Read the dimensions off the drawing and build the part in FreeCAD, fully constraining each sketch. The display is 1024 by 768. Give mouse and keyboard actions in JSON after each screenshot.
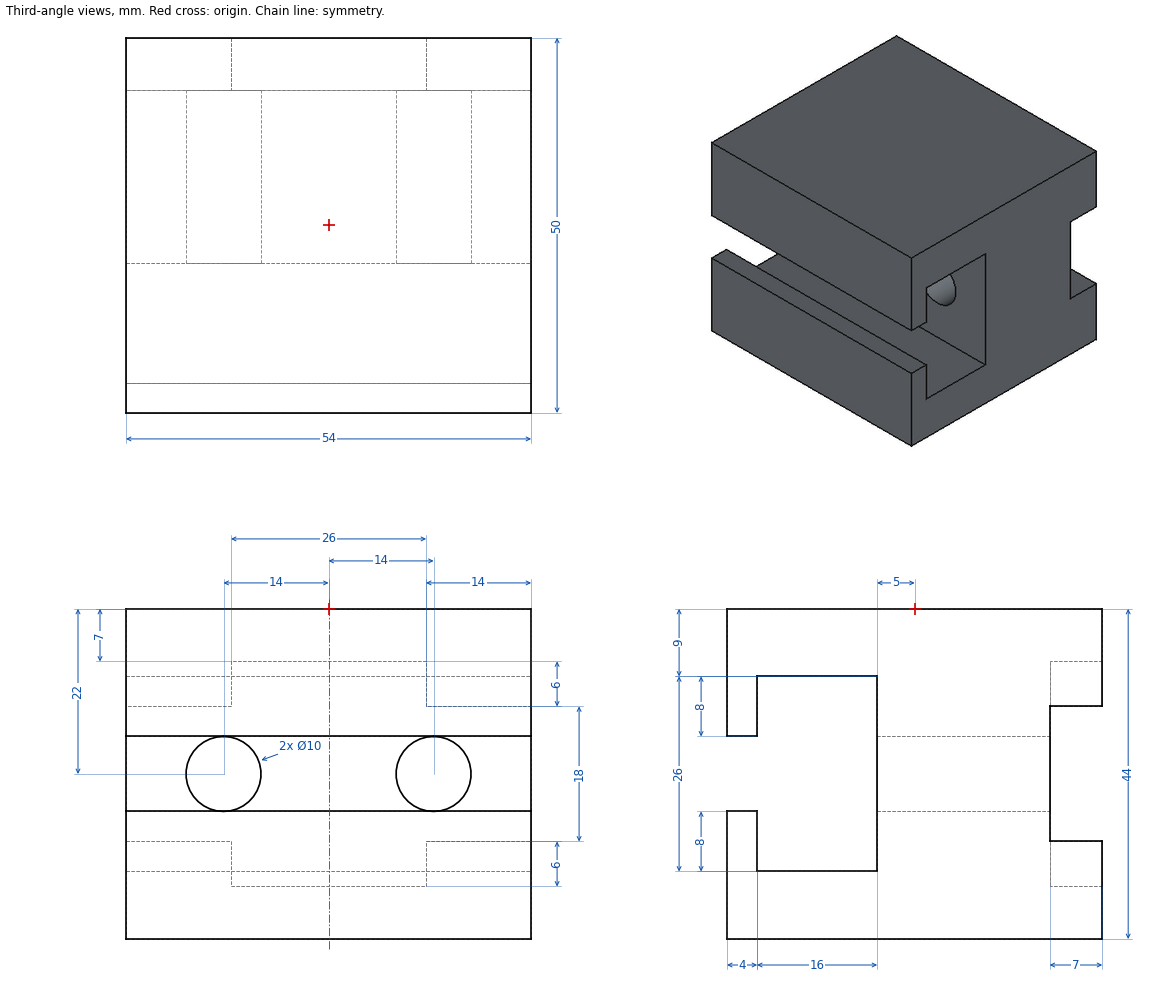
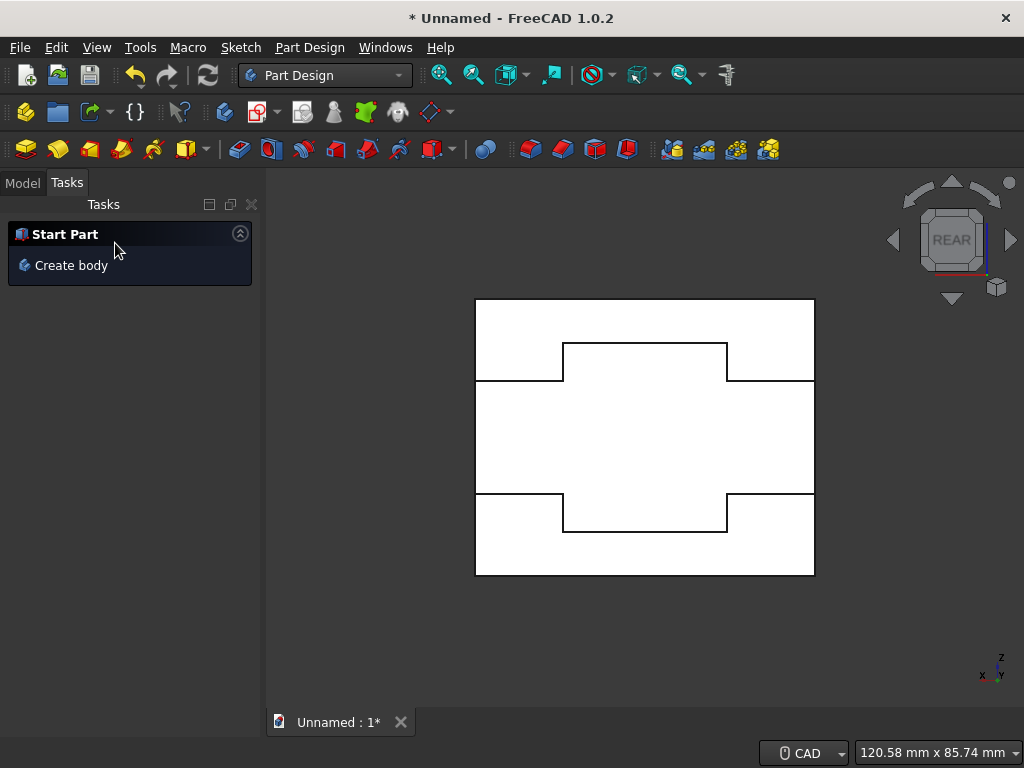
{"action": "key", "text": "6"}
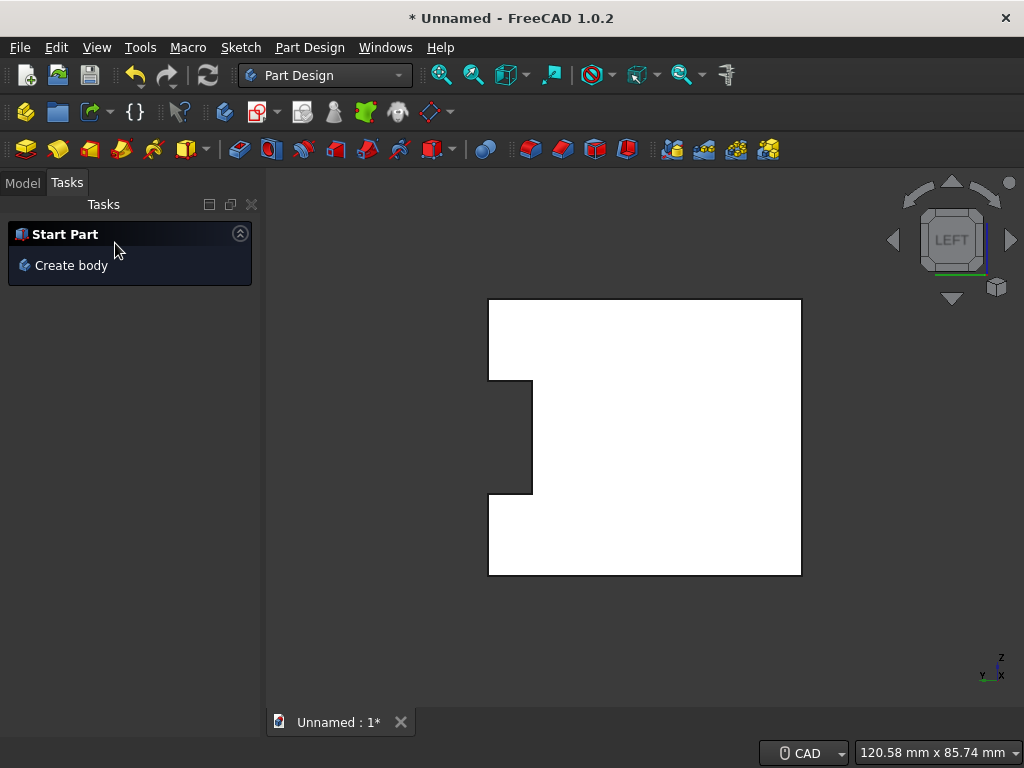
{"action": "left_click", "coordinate": [645, 437]}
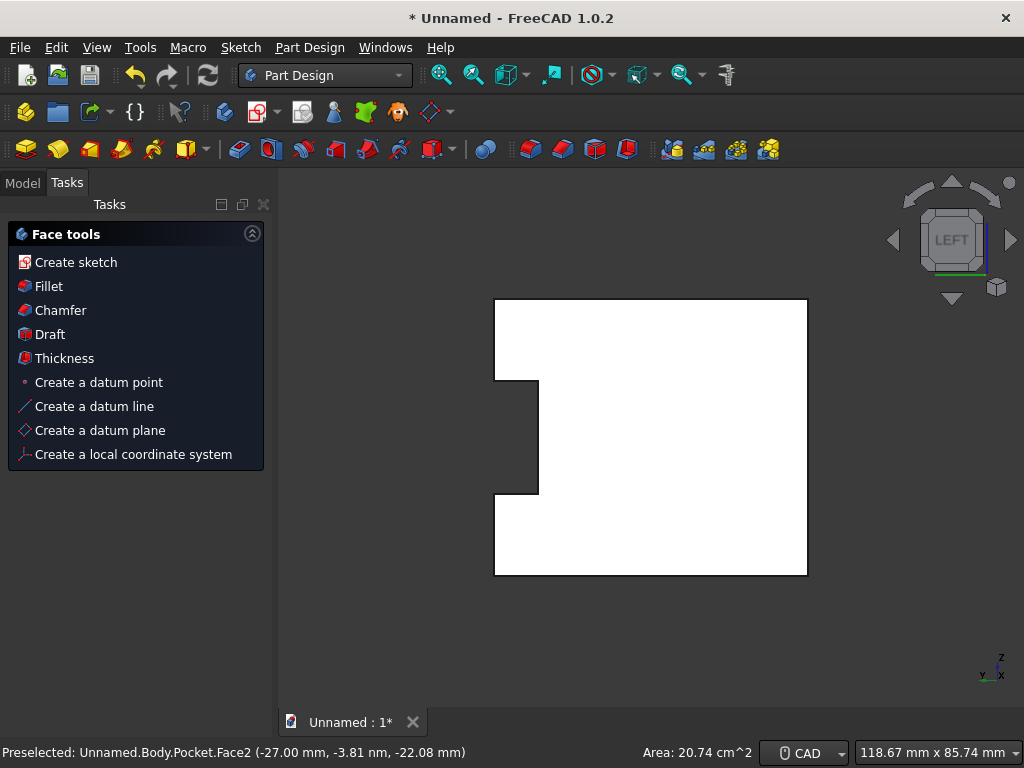
{"action": "left_click", "coordinate": [258, 112]}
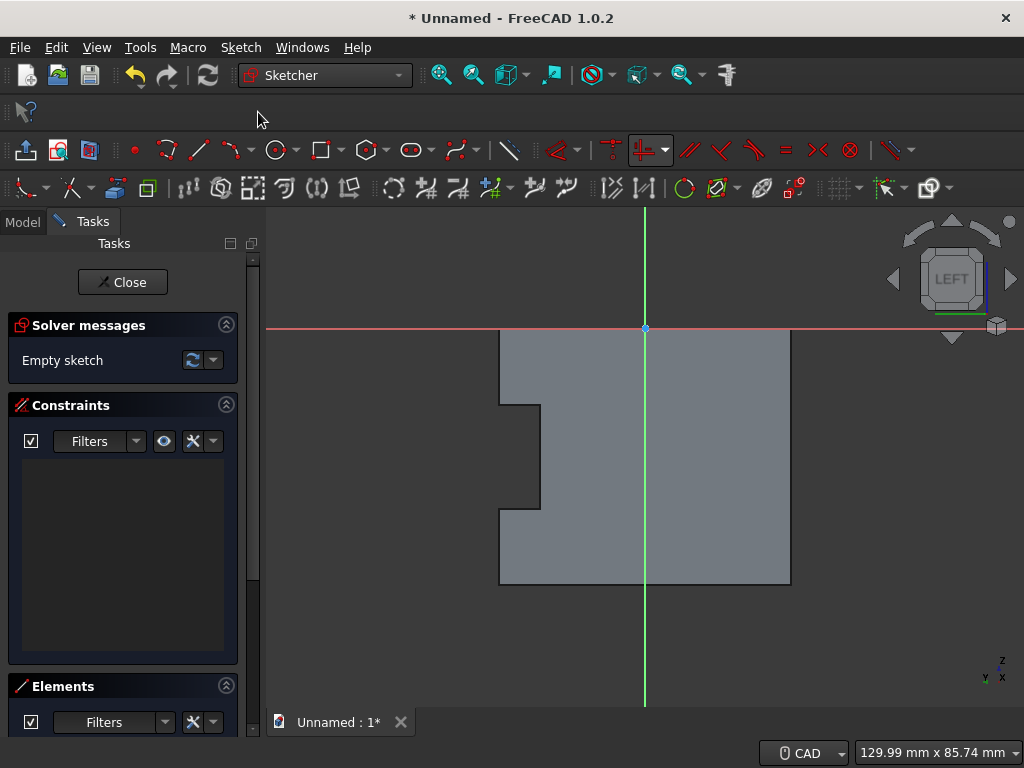
{"action": "scroll", "coordinate": [859, 377], "scroll_direction": "up", "scroll_amount": 2}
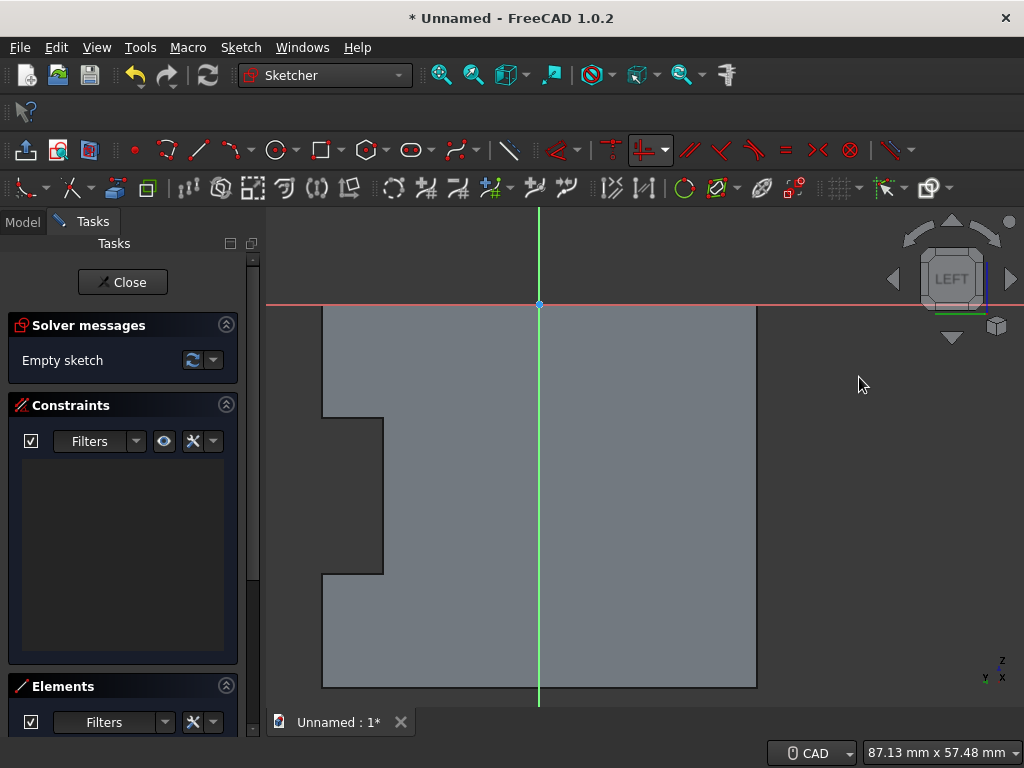
{"action": "left_click", "coordinate": [168, 150]}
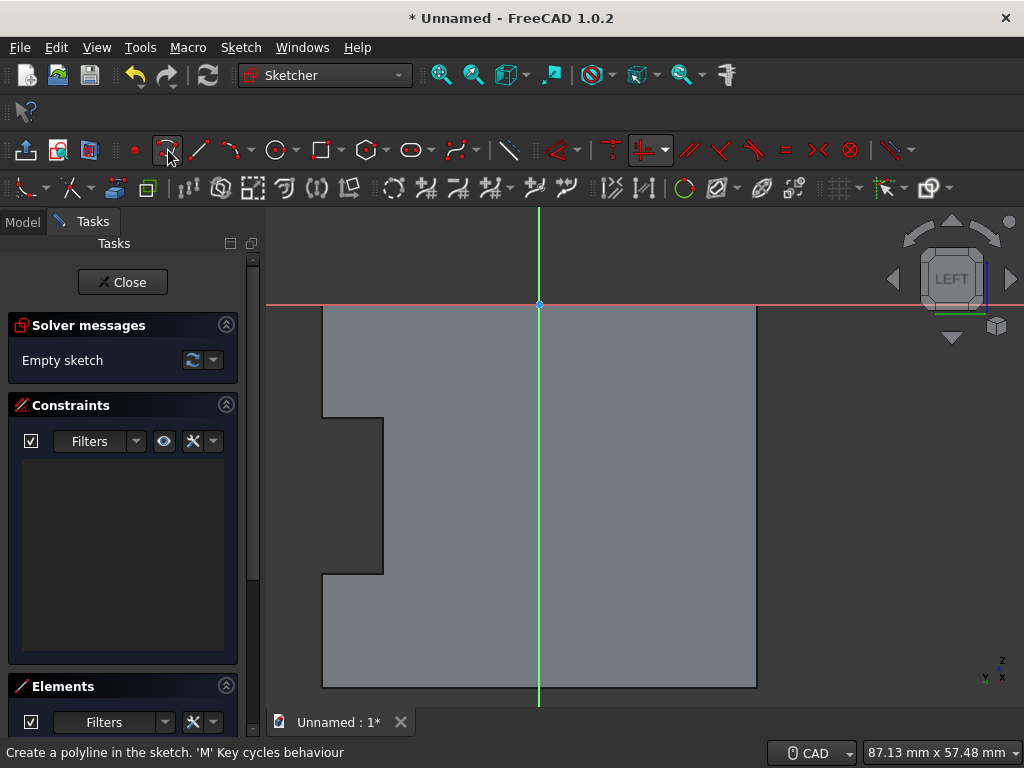
{"action": "left_click", "coordinate": [583, 383]}
{"action": "left_click", "coordinate": [583, 609]}
{"action": "left_click", "coordinate": [722, 609]}
{"action": "left_click", "coordinate": [722, 540]}
{"action": "left_click", "coordinate": [757, 540]}
{"action": "left_click", "coordinate": [757, 453]}
{"action": "left_click", "coordinate": [722, 453]}
{"action": "left_click", "coordinate": [722, 383]}
{"action": "left_click", "coordinate": [583, 384]}
{"action": "key", "text": "Escape"}
{"action": "key", "text": "Escape"}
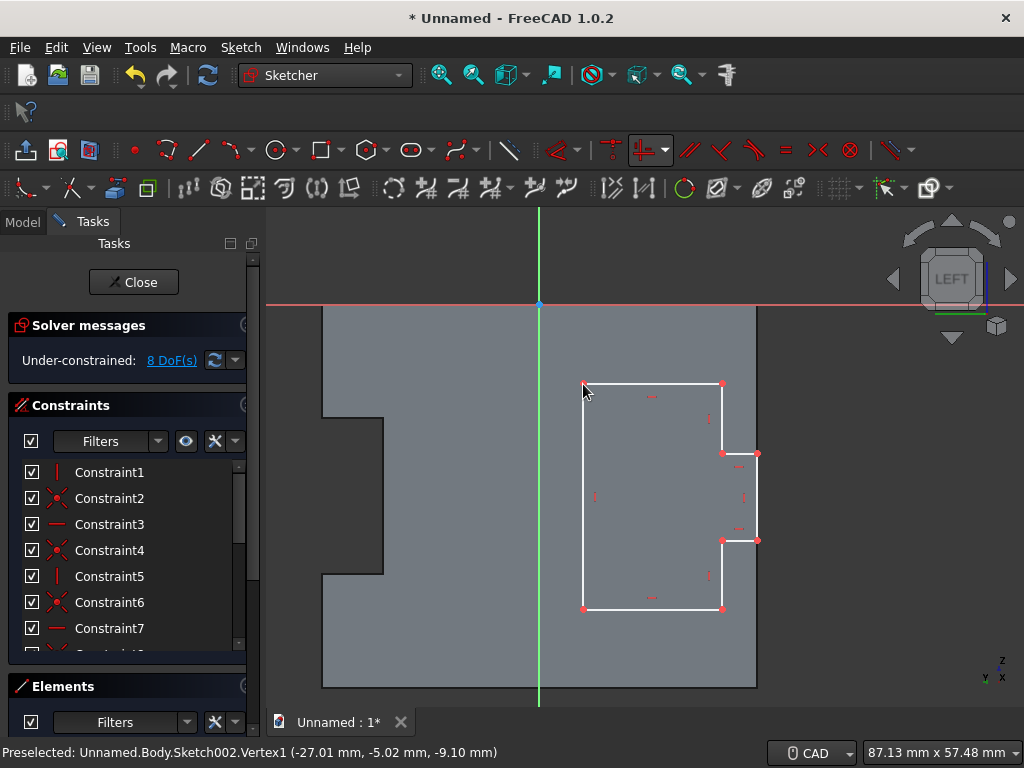
{"action": "key", "text": "d"}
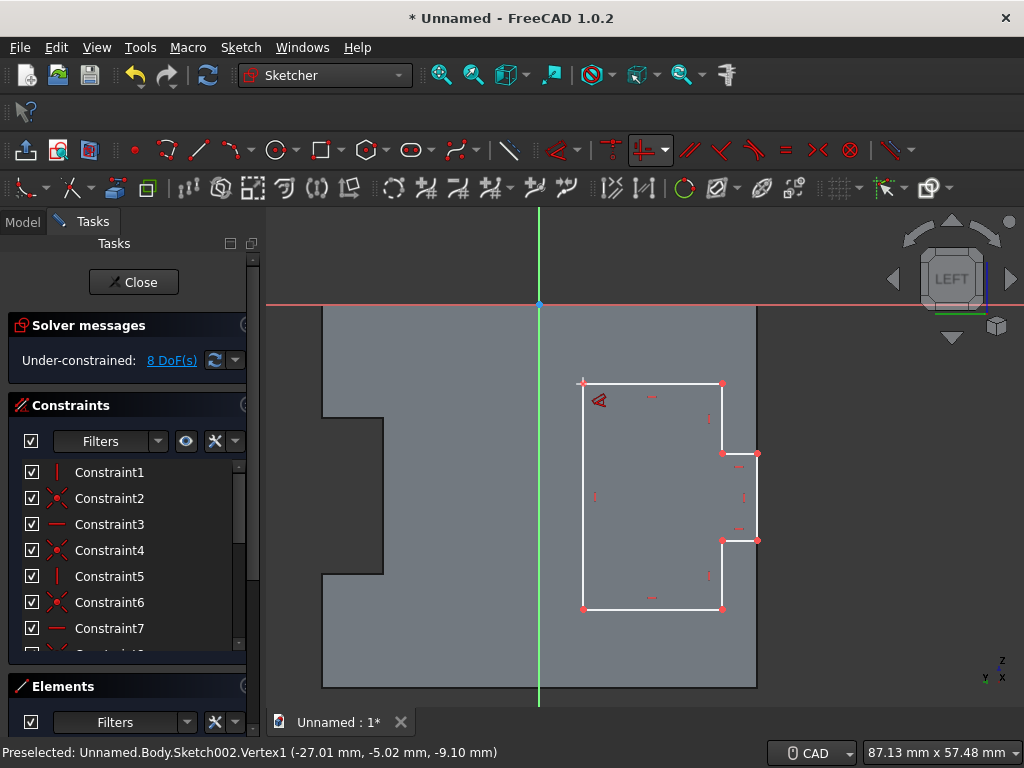
{"action": "left_click", "coordinate": [722, 589]}
{"action": "left_click", "coordinate": [756, 575]}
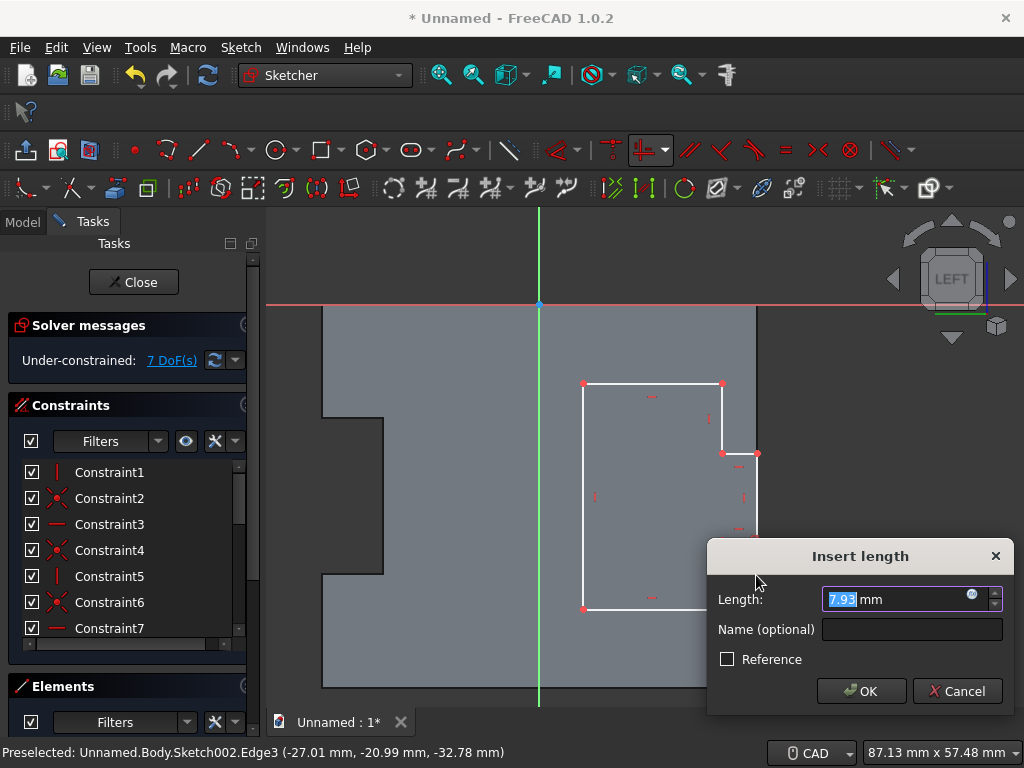
{"action": "type", "text": "8"}
{"action": "key", "text": "Return"}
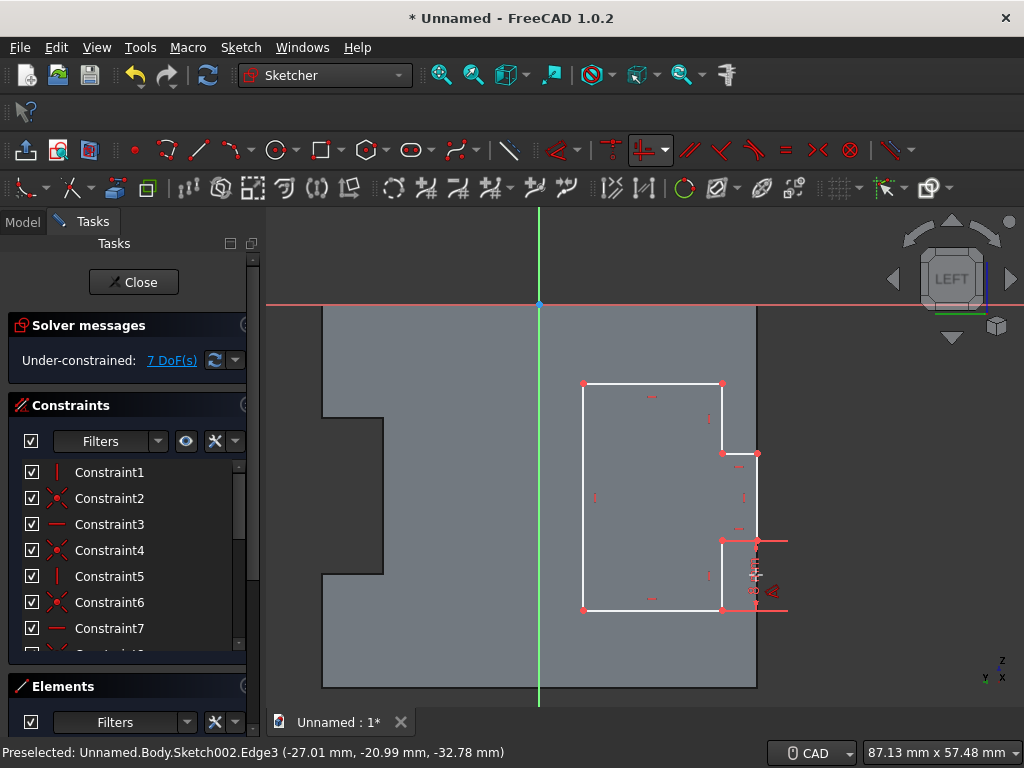
{"action": "scroll", "coordinate": [733, 541], "scroll_direction": "up", "scroll_amount": 2}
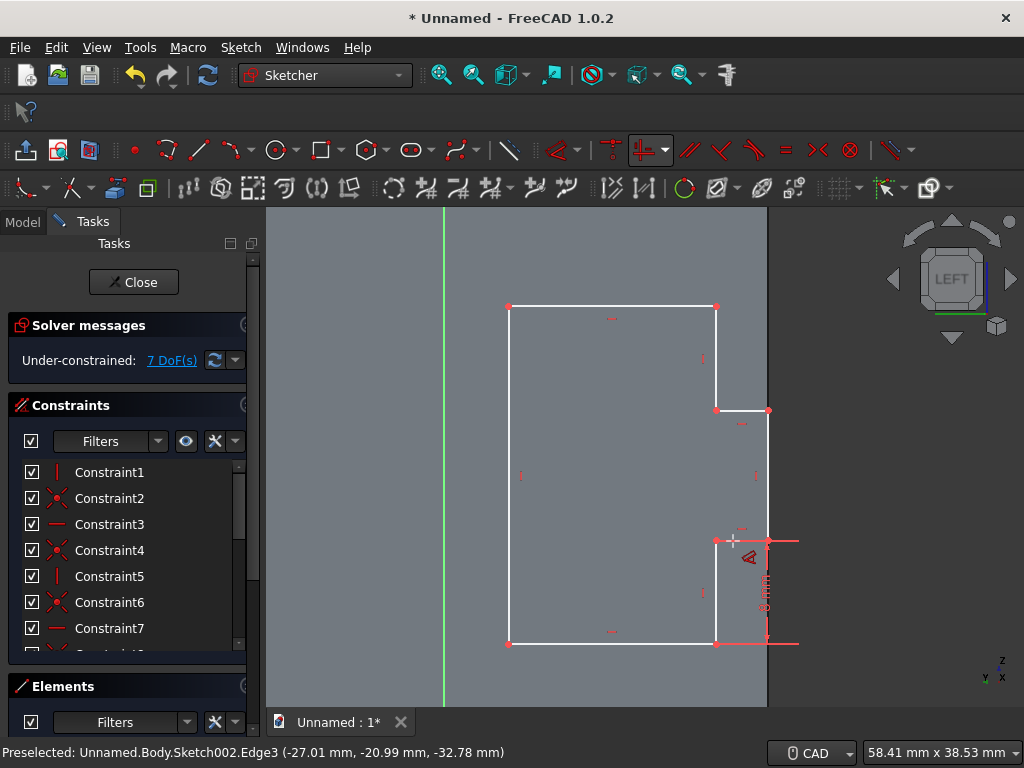
{"action": "left_click", "coordinate": [732, 541]}
{"action": "left_click", "coordinate": [742, 507]}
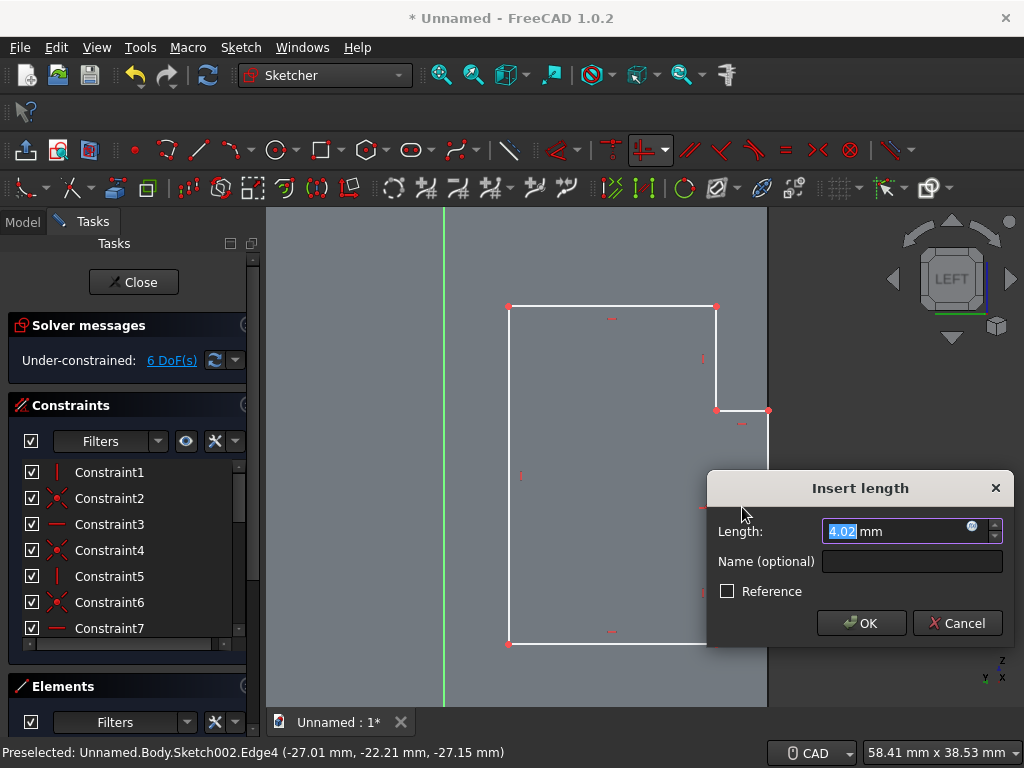
{"action": "type", "text": "4"}
{"action": "key", "text": "Return"}